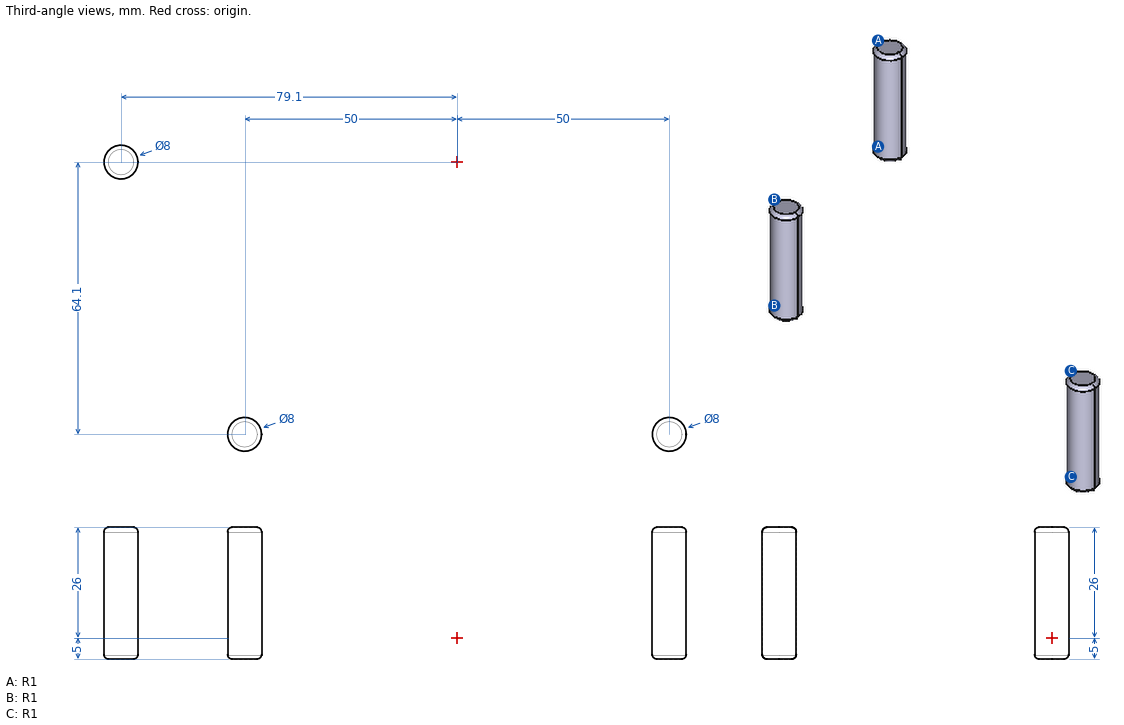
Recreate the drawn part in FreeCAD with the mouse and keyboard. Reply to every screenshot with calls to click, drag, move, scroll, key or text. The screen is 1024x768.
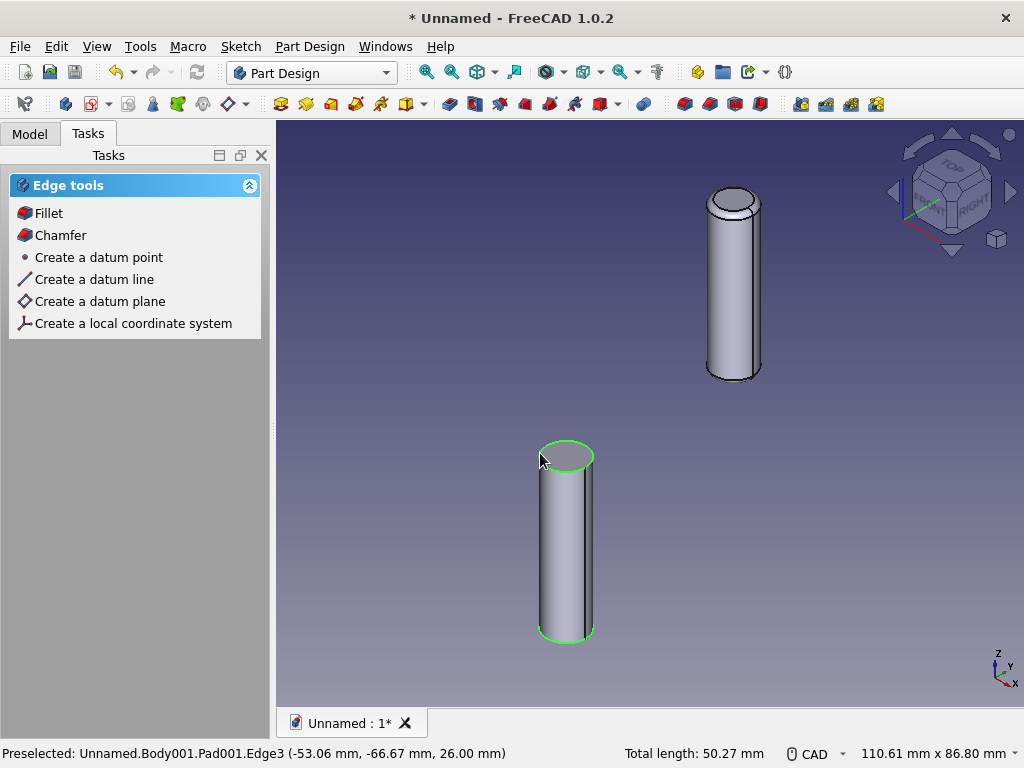
click(685, 104)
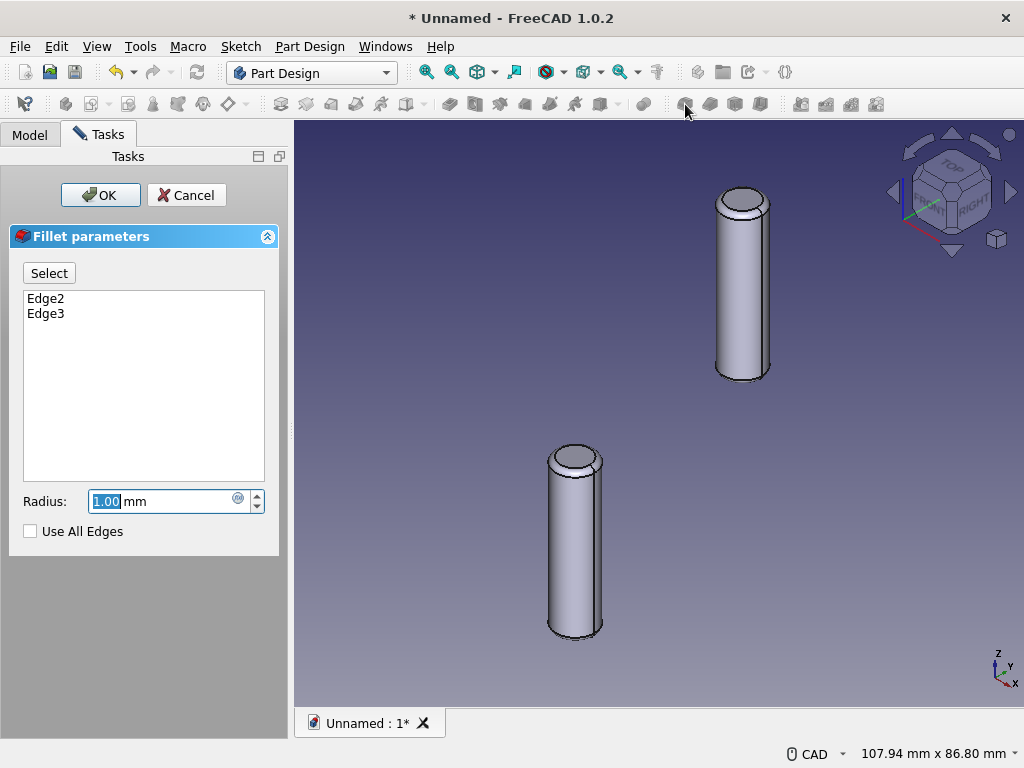
text(1)
key(Tab)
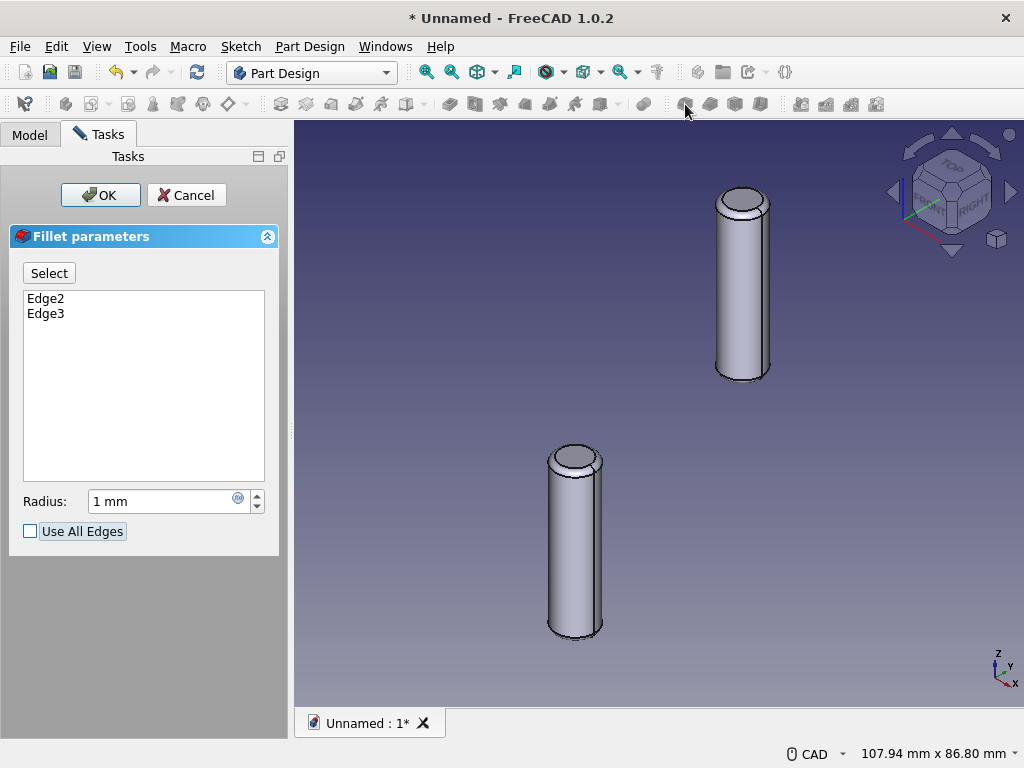
click(101, 195)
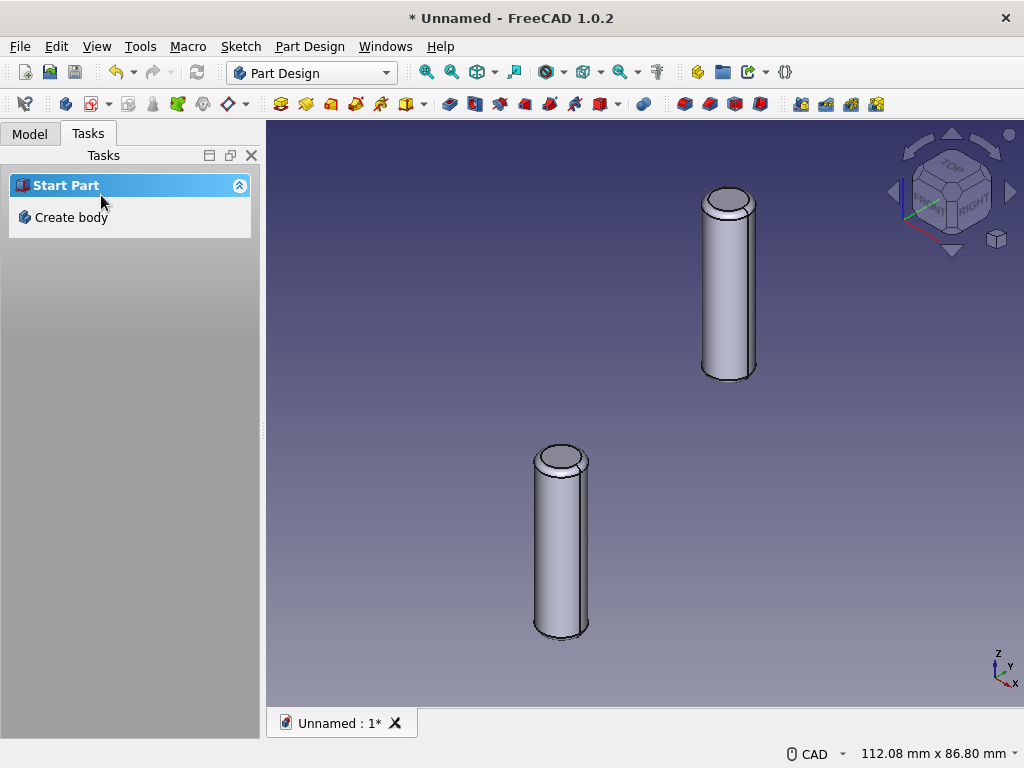
click(427, 72)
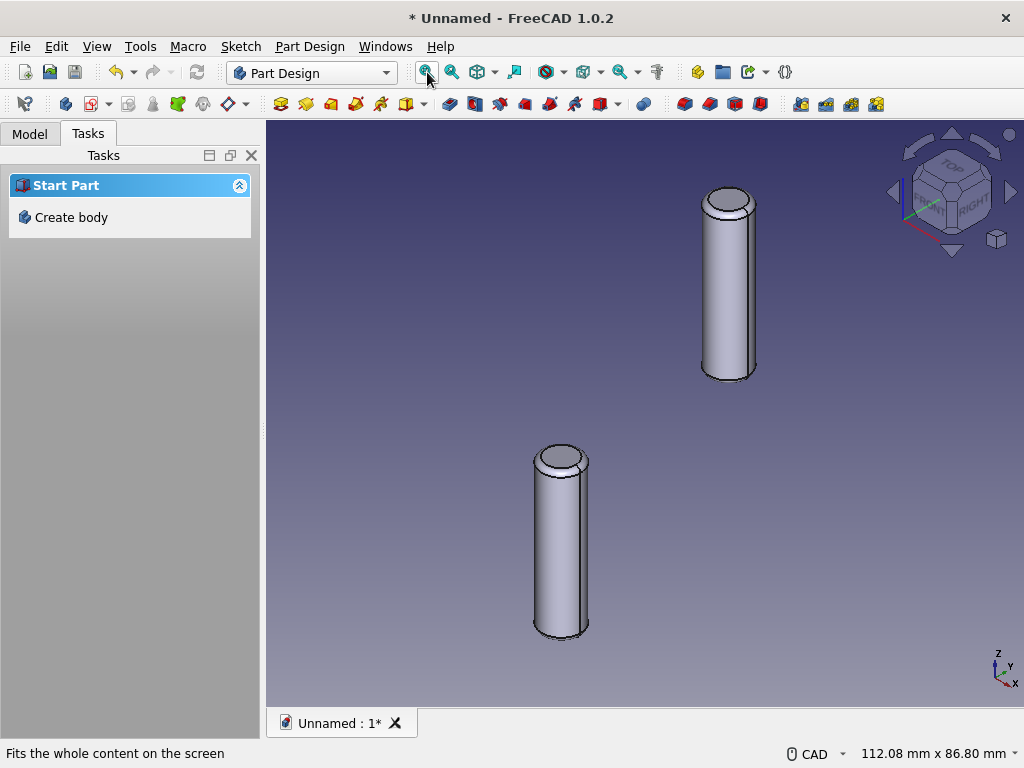
click(66, 104)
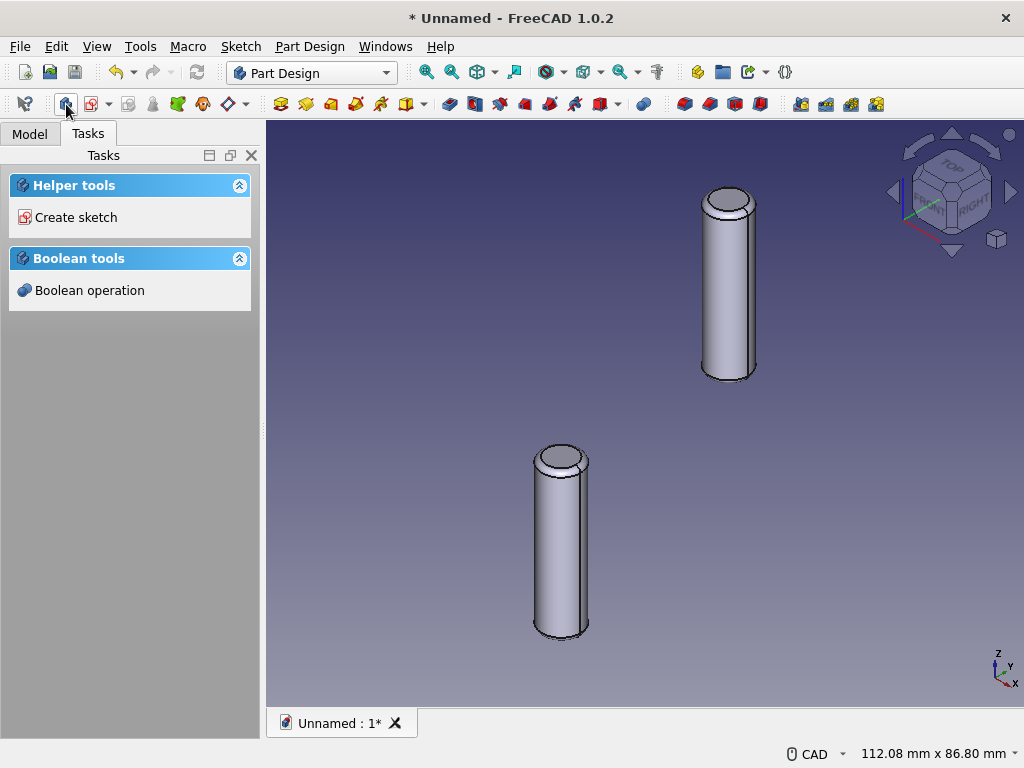
click(306, 667)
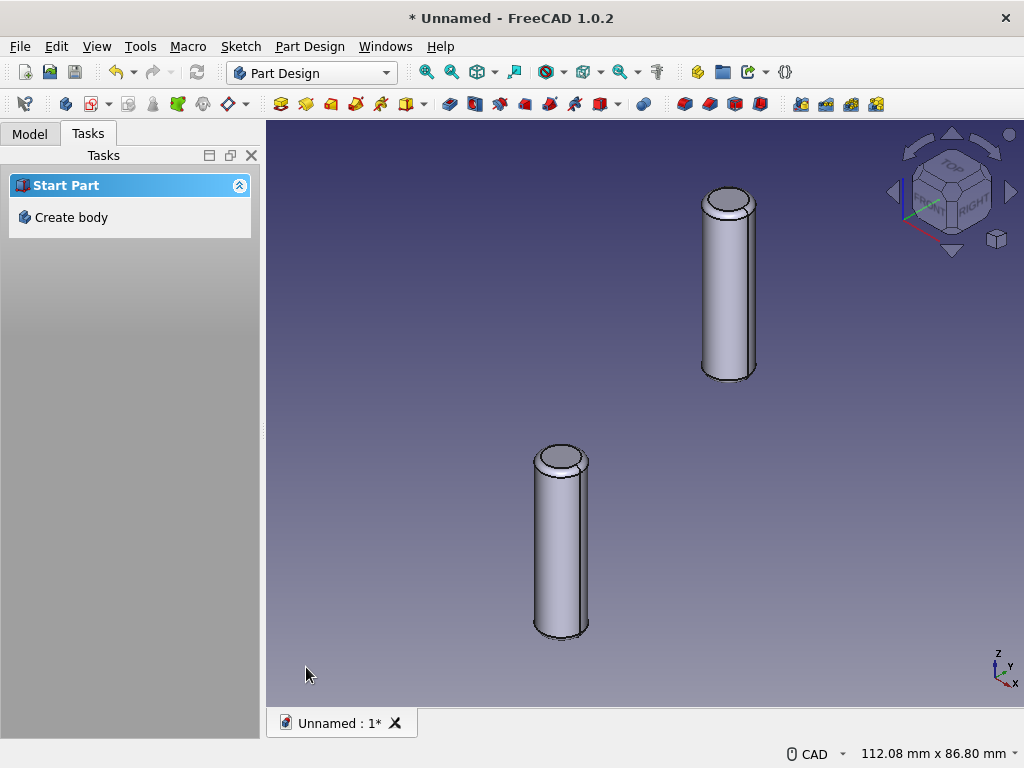
click(90, 104)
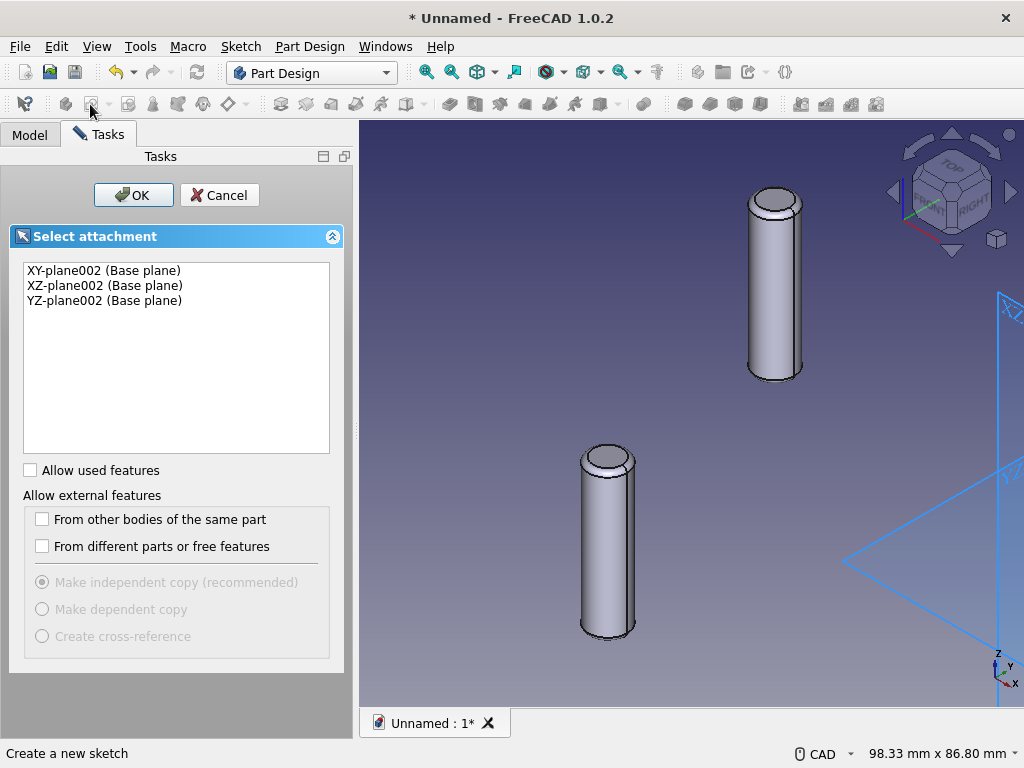
click(84, 270)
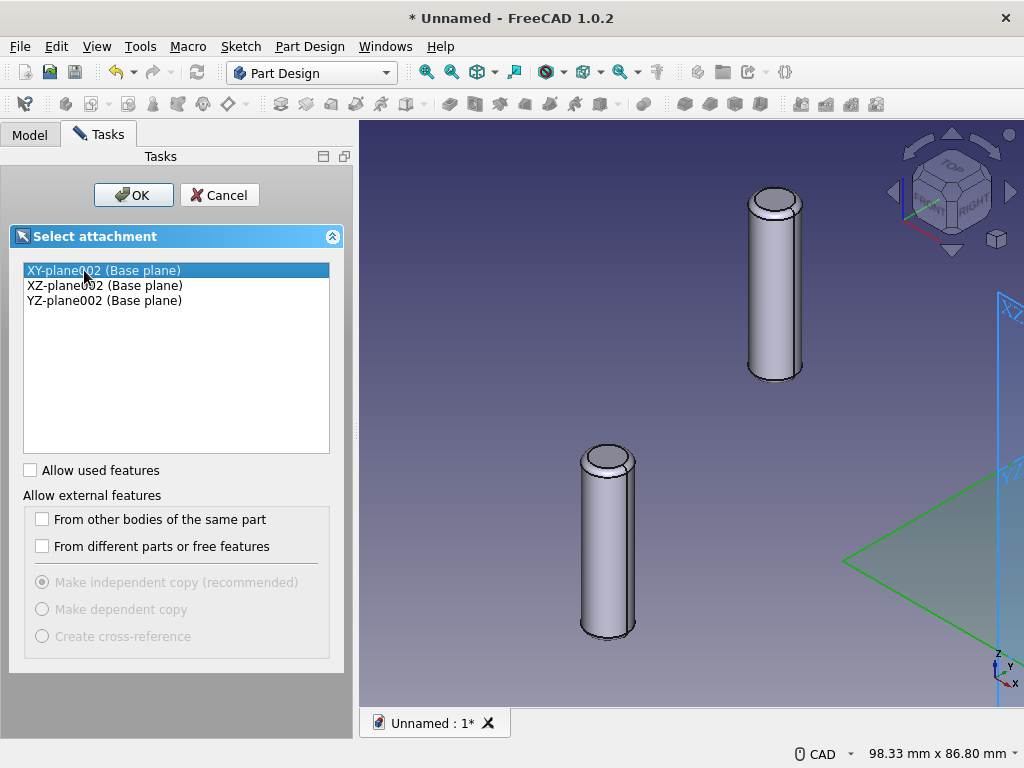
click(134, 195)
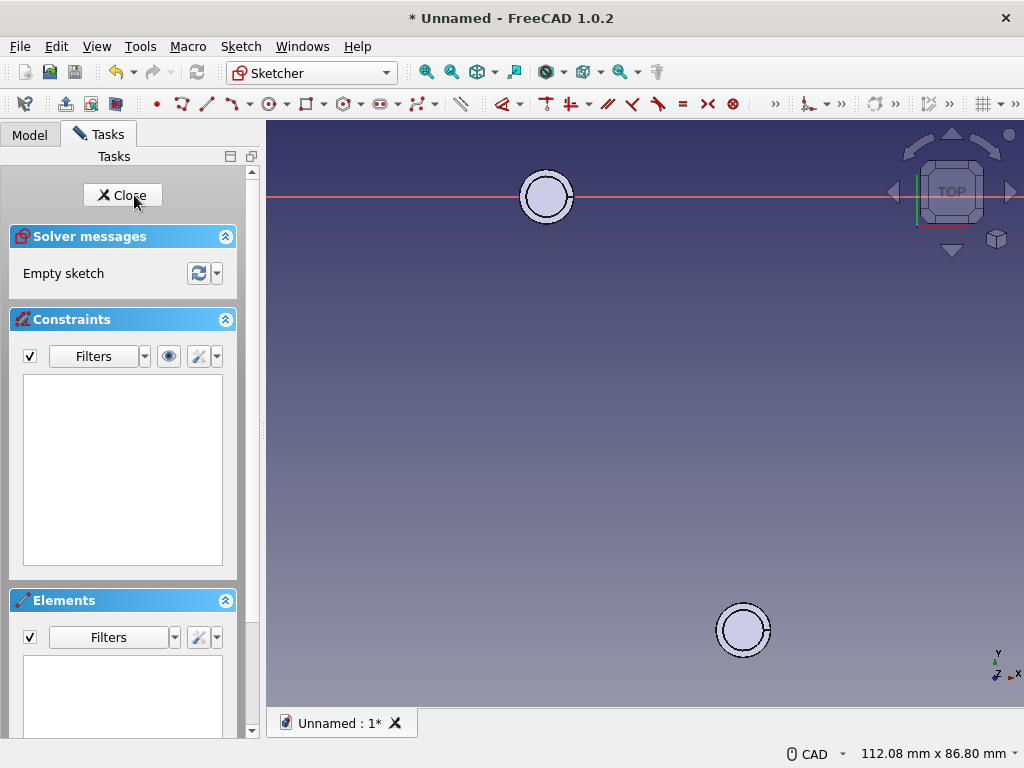
scroll(576, 414, down, 5)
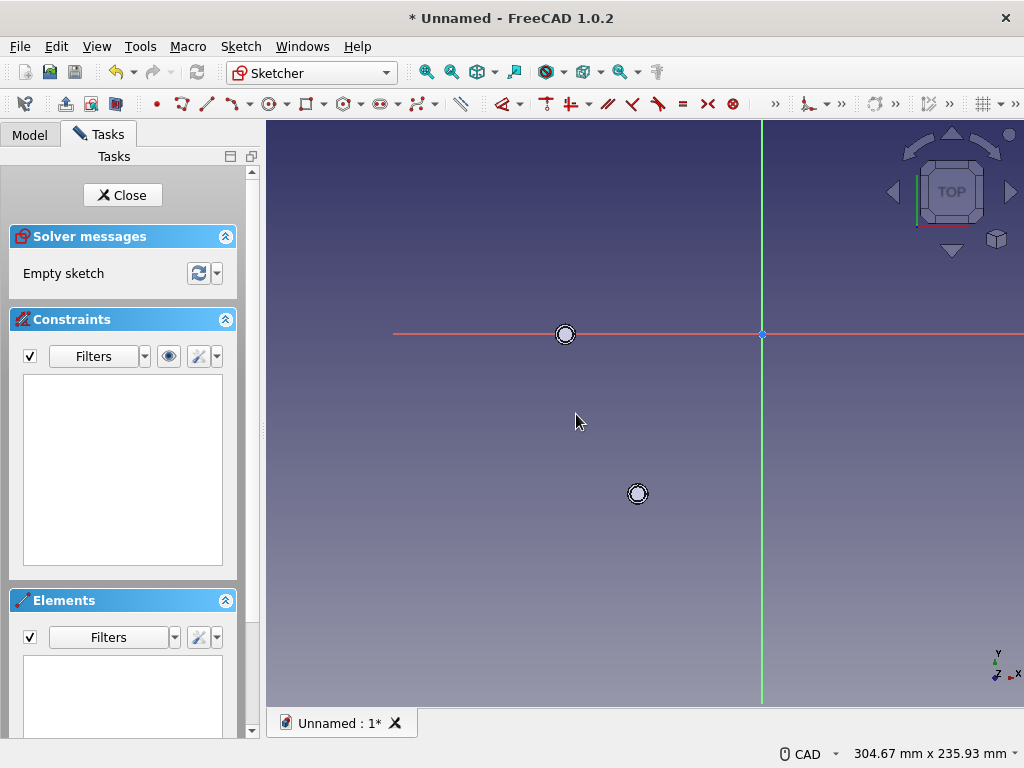
scroll(576, 414, down, 5)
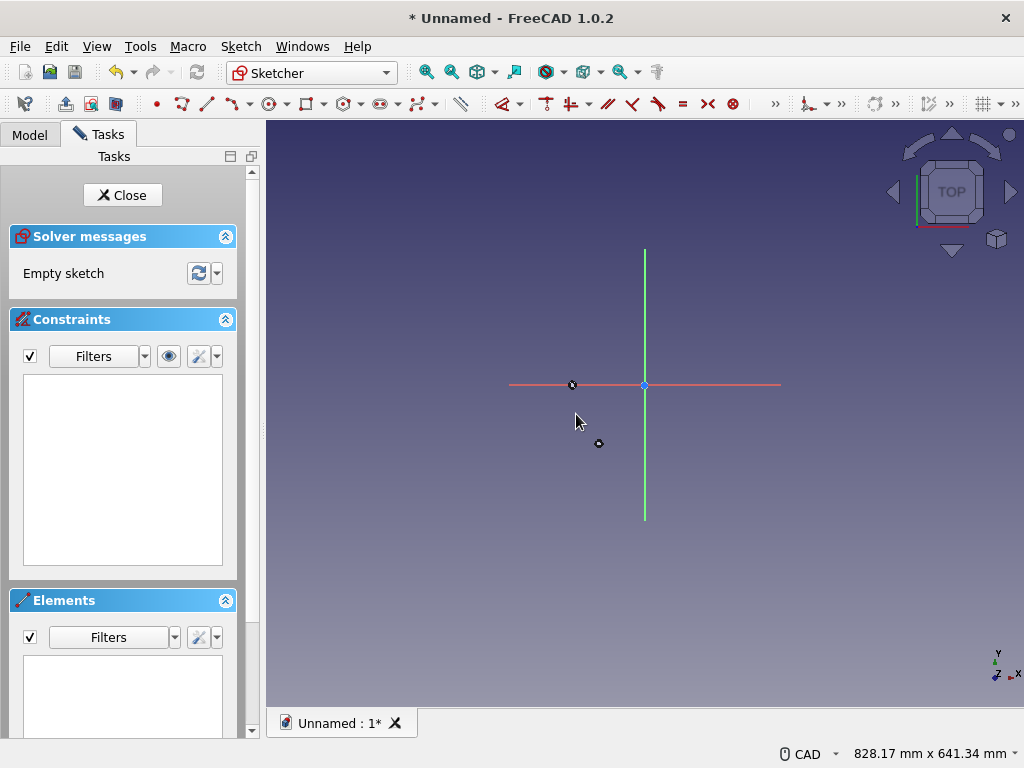
scroll(697, 445, up, 15)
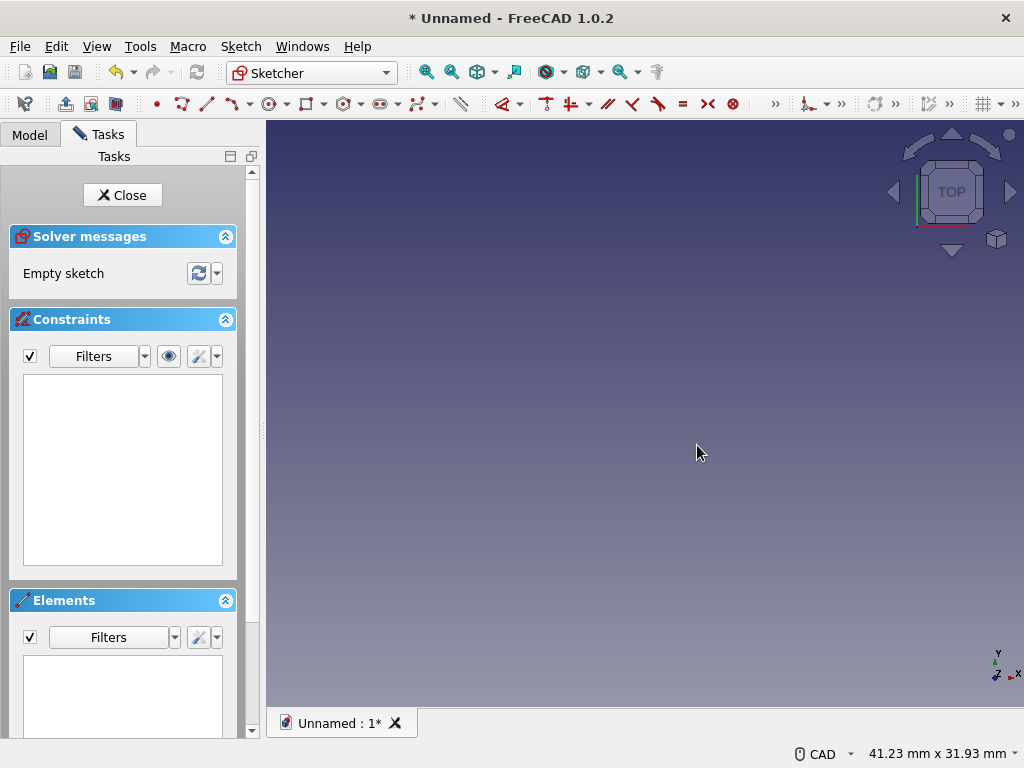
scroll(544, 405, up, 5)